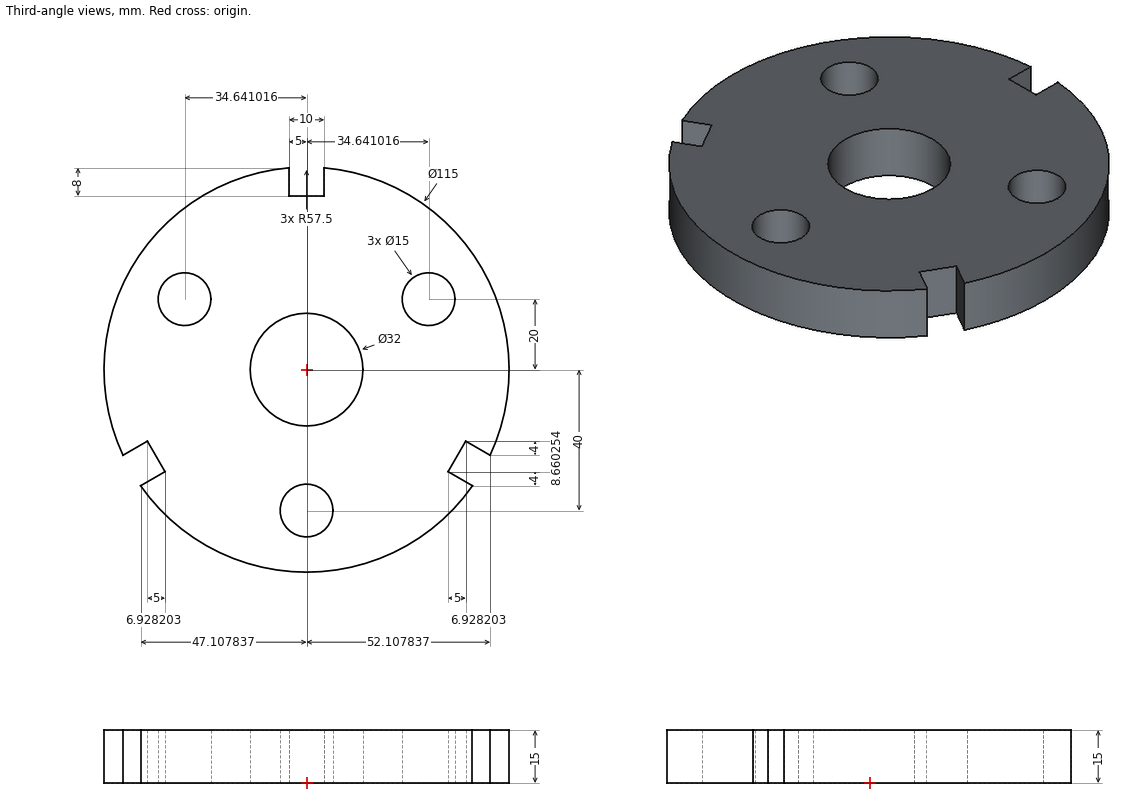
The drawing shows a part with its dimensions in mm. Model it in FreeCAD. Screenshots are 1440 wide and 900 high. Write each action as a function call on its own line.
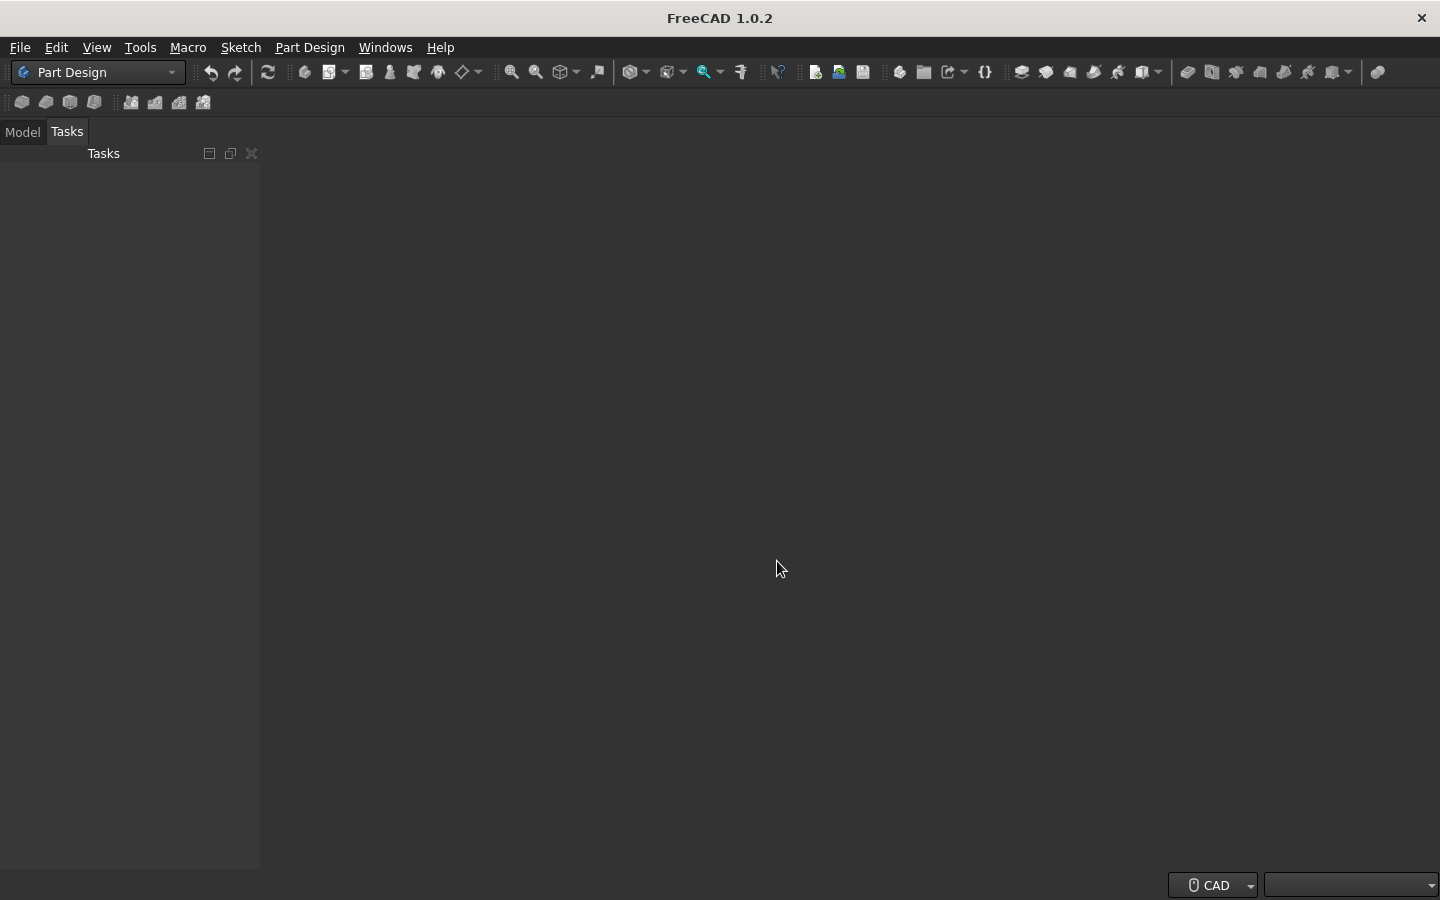
click(816, 72)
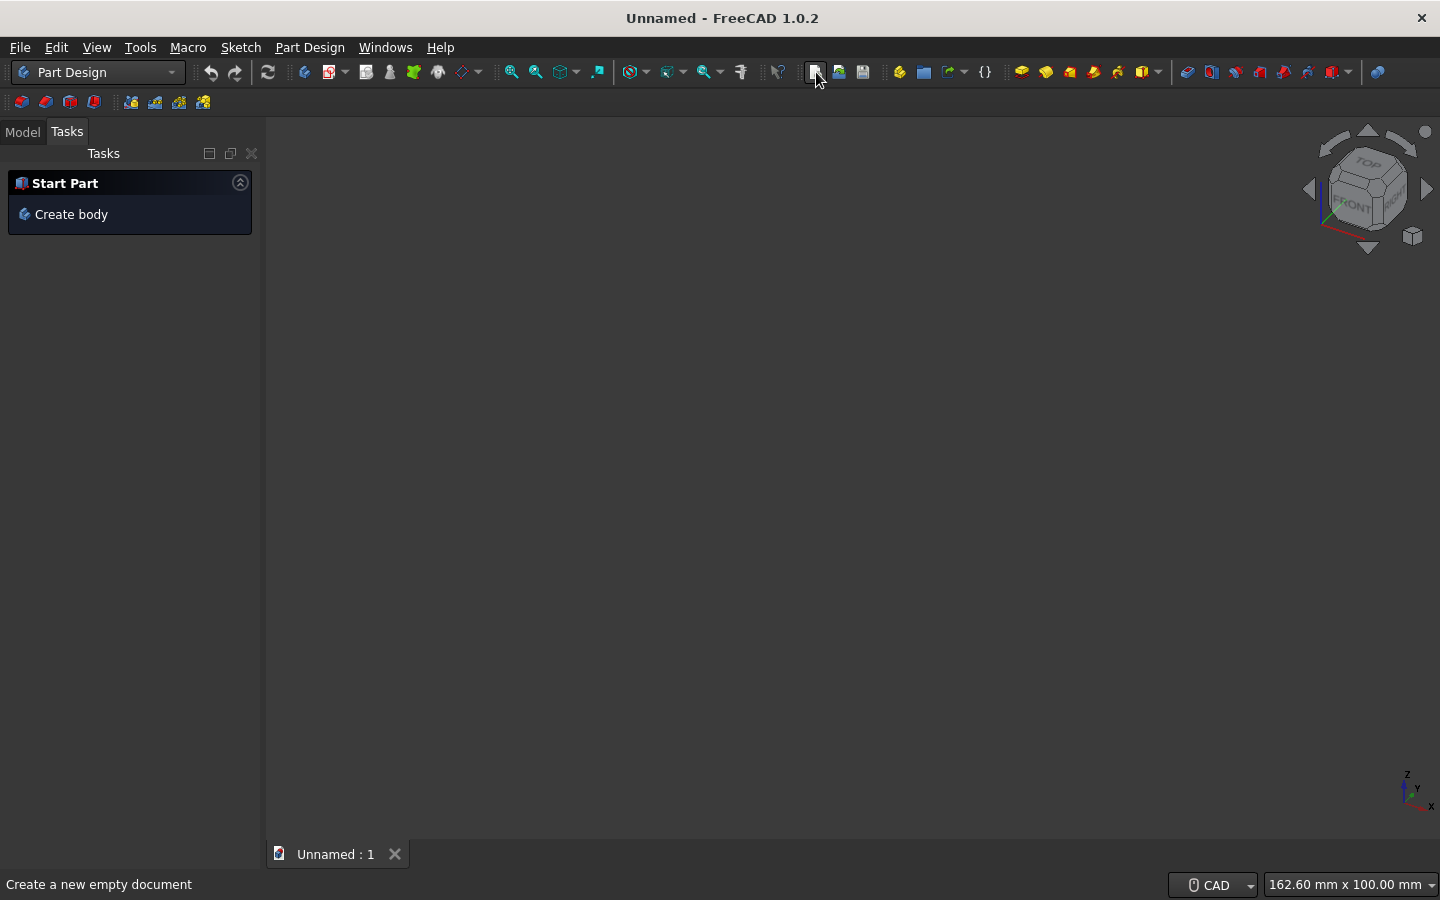
click(330, 72)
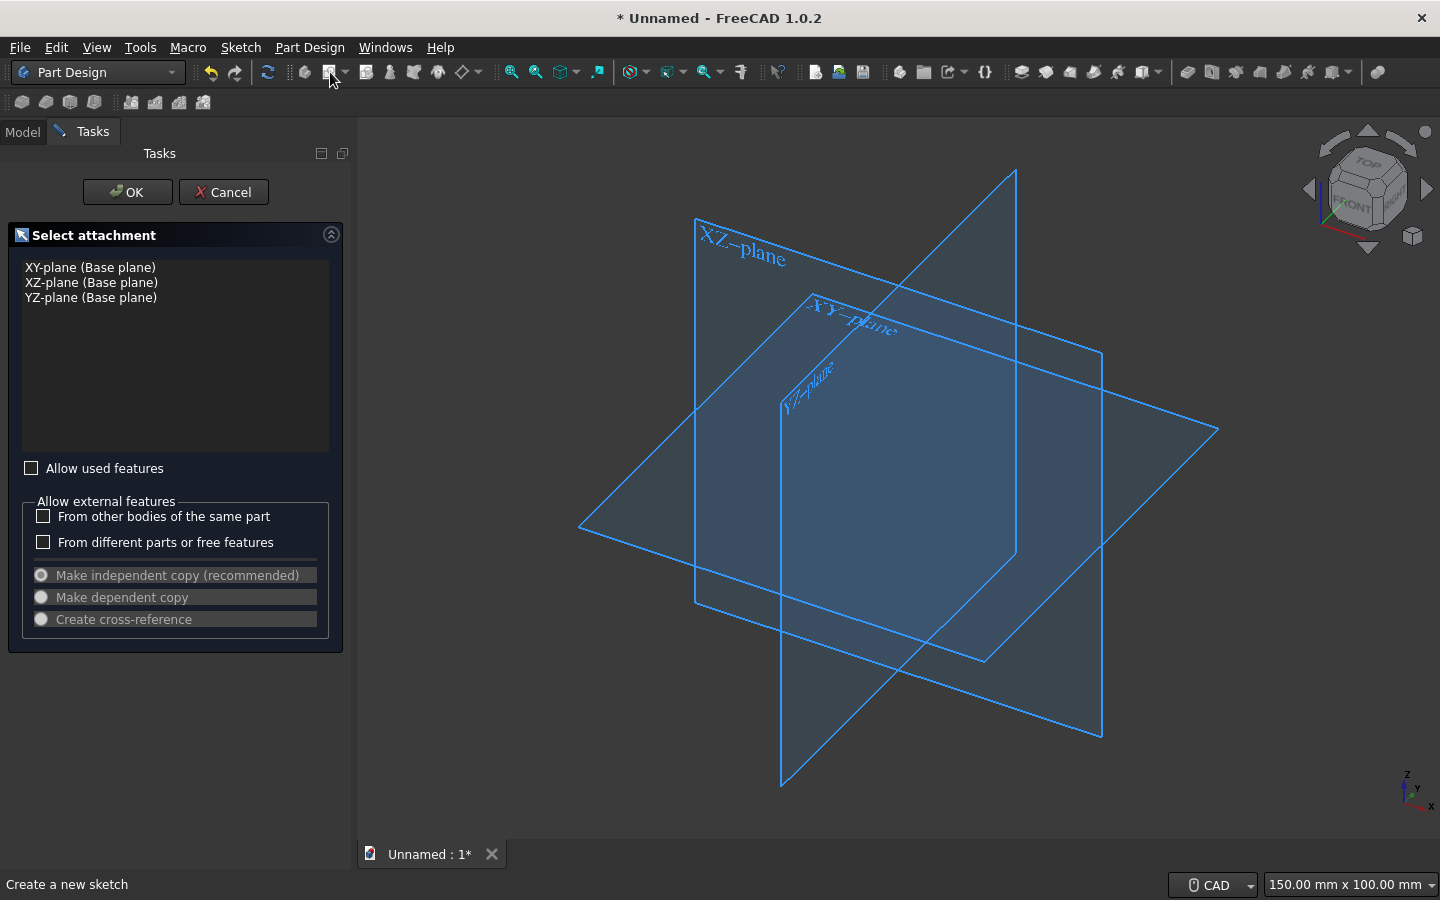
click(82, 268)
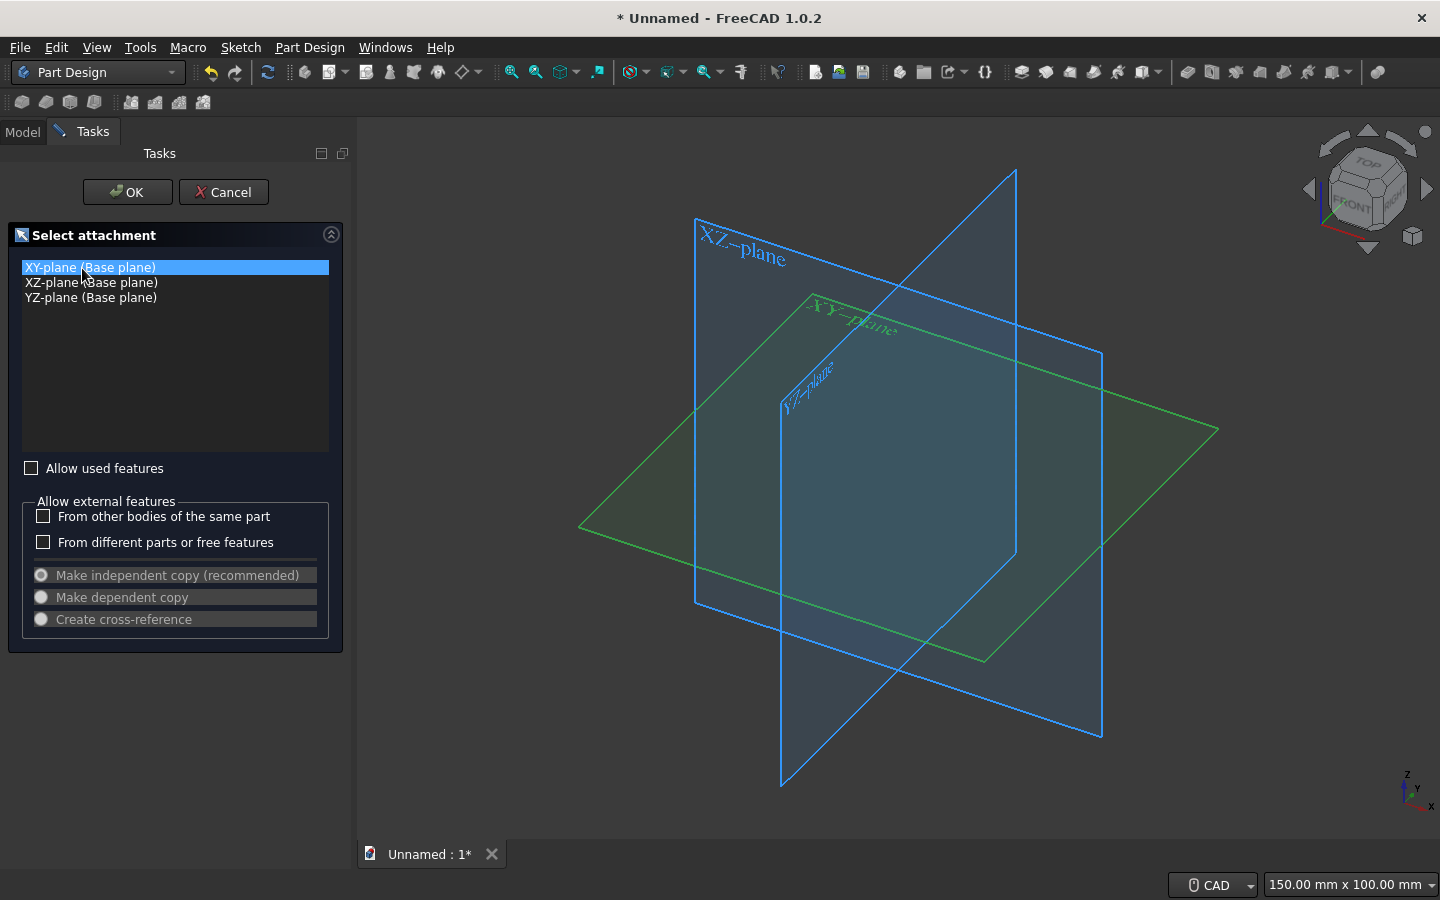
click(128, 192)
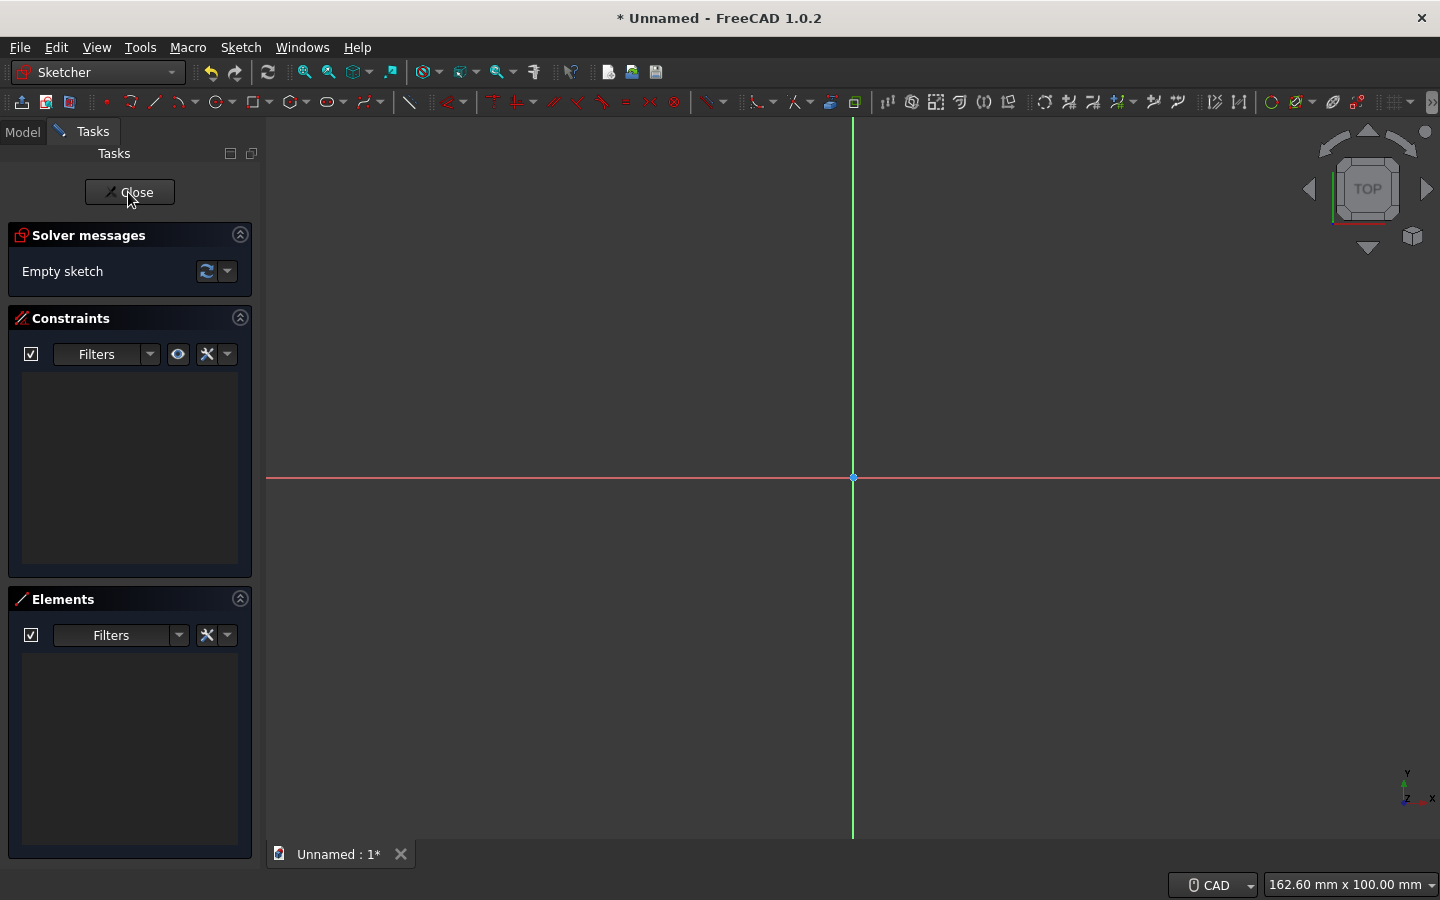
scroll(701, 478, down, 3)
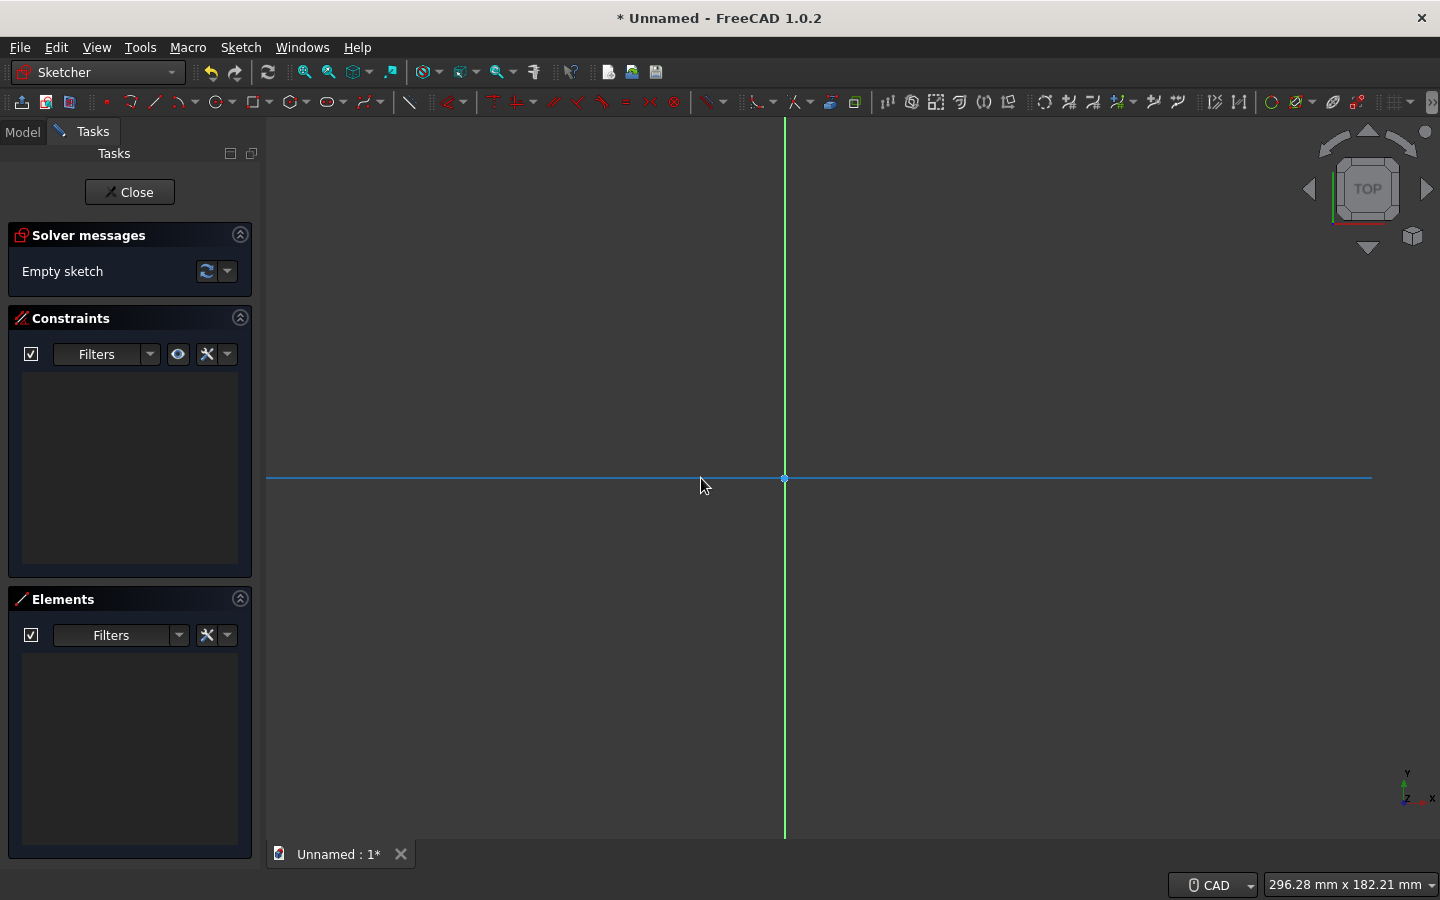
click(216, 102)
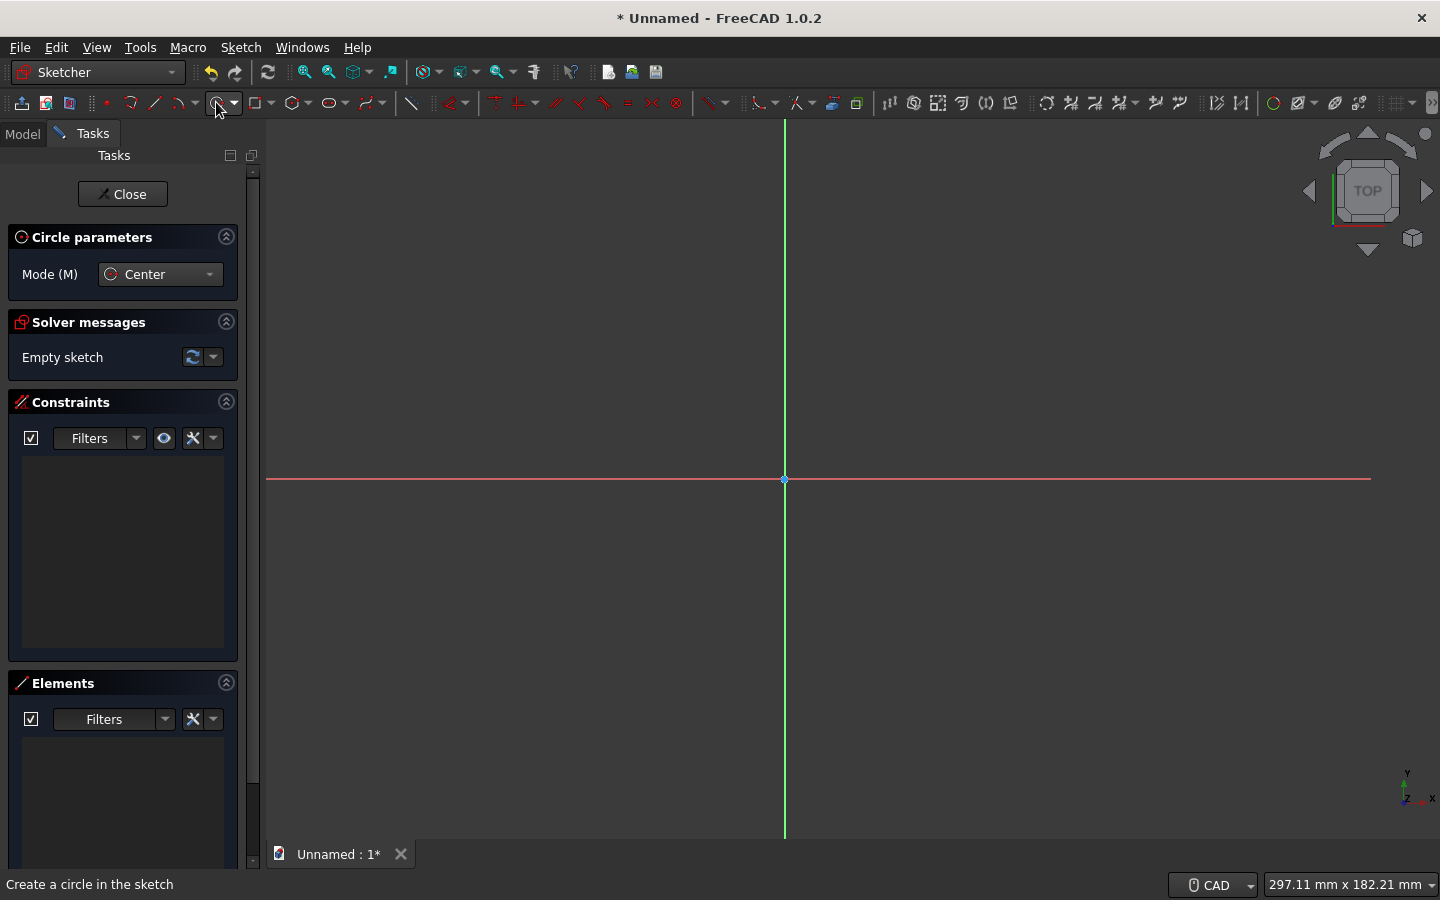
click(785, 479)
move(945, 319)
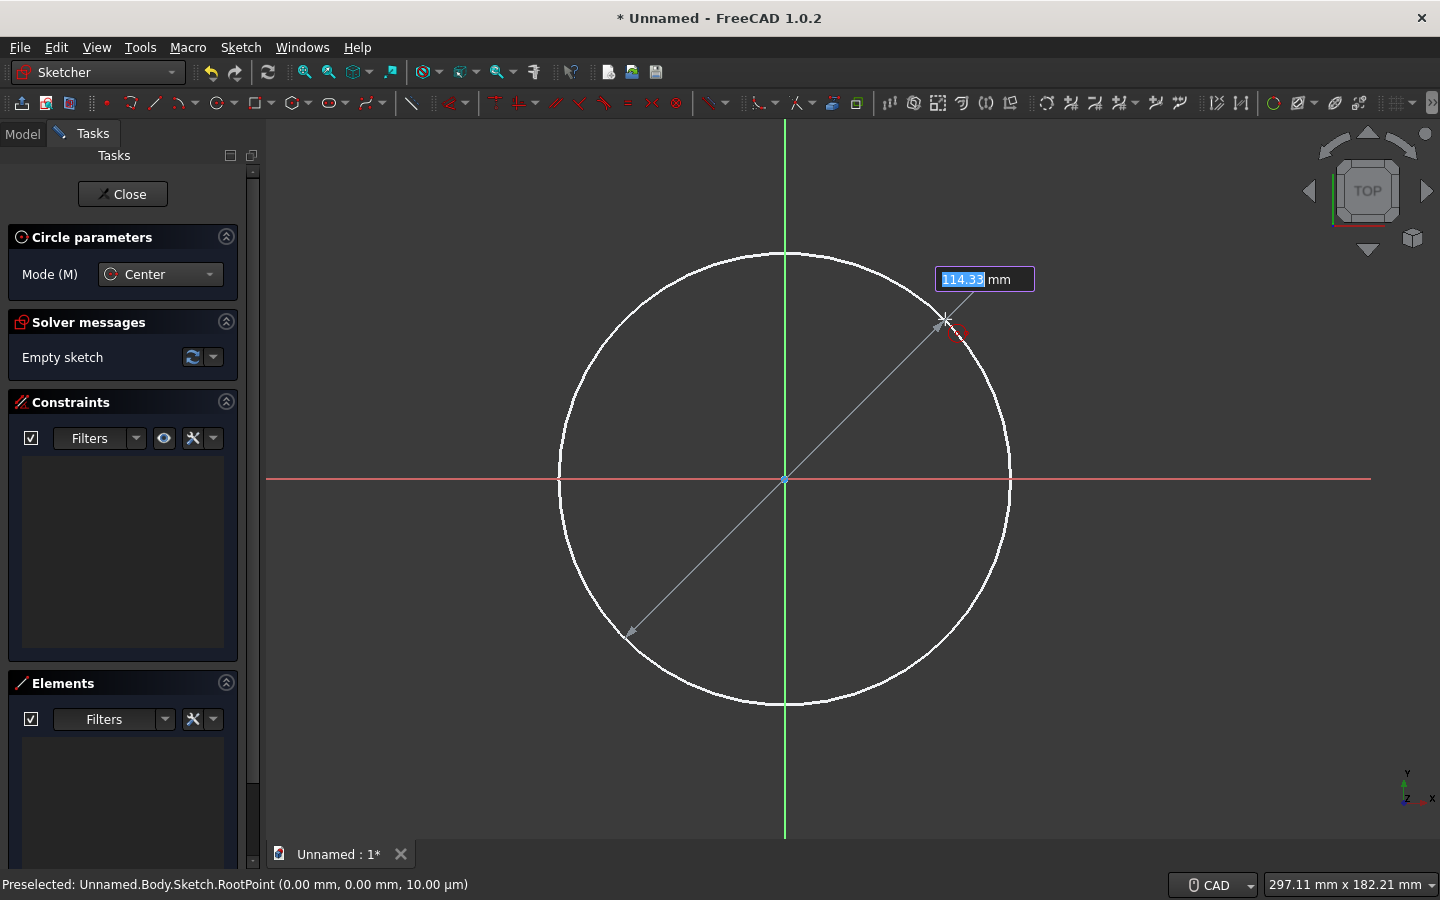
text(115)
key(Return)
key(Escape)